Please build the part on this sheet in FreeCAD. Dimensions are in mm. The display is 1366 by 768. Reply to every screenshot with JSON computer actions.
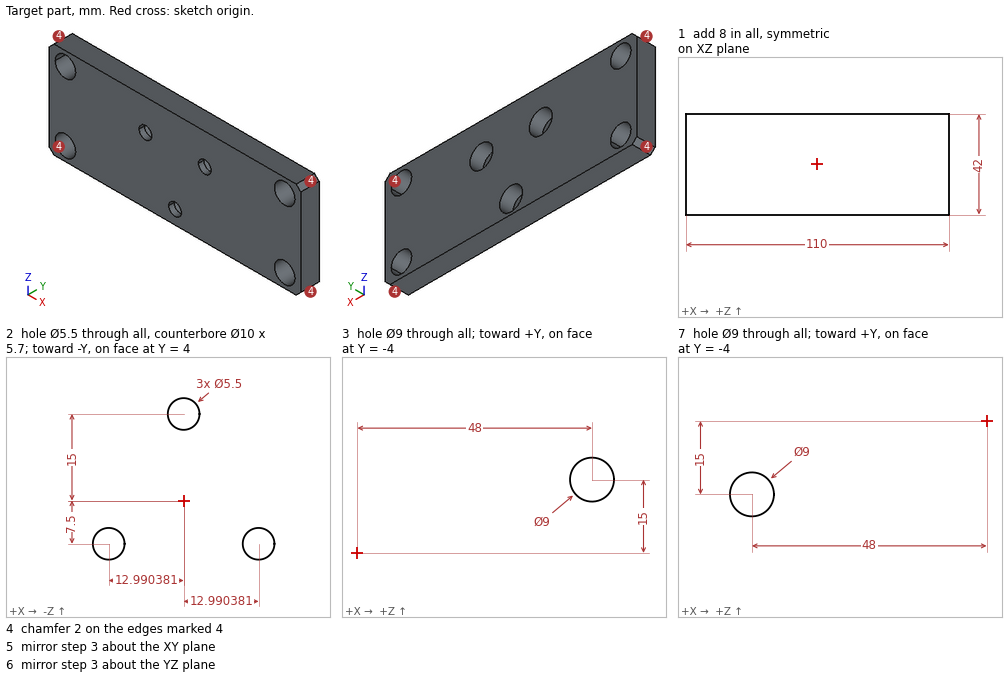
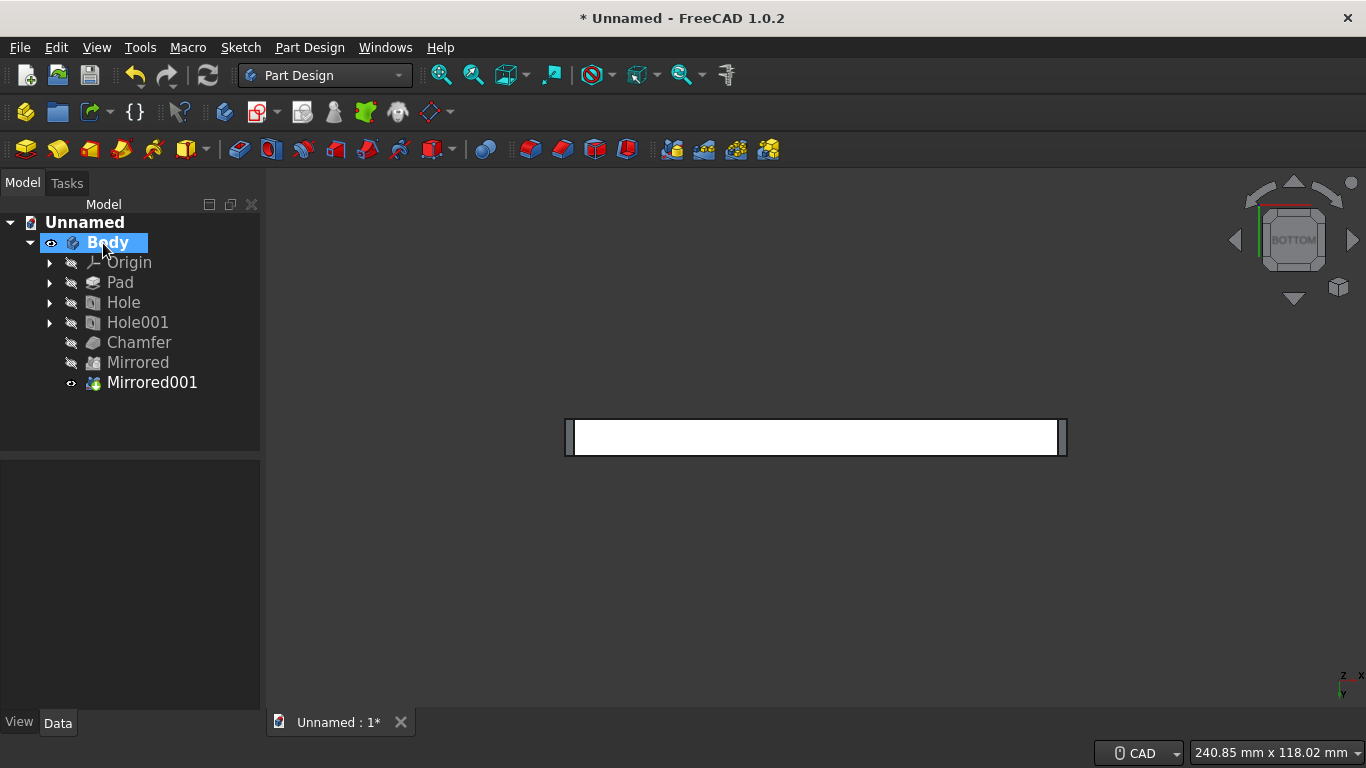
{"action": "key", "text": "0"}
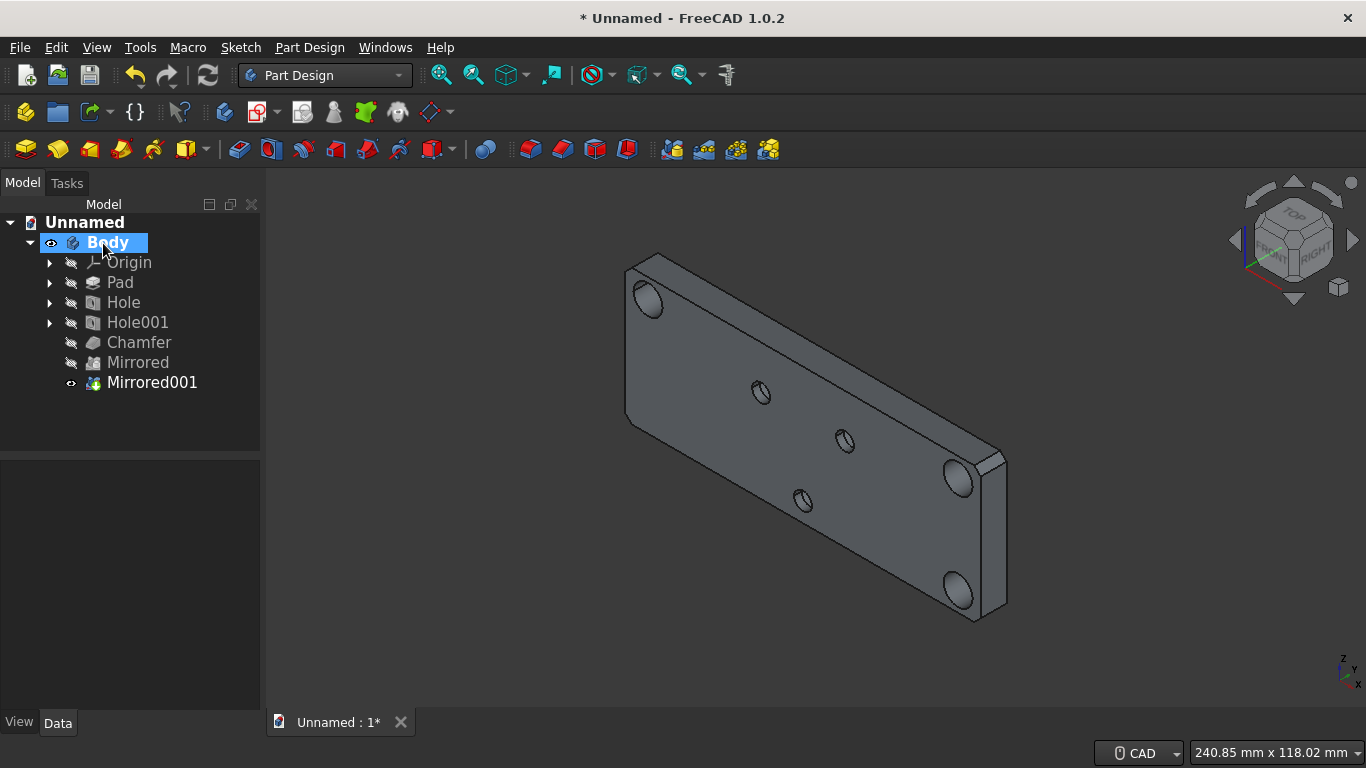
{"action": "left_click", "coordinate": [905, 503]}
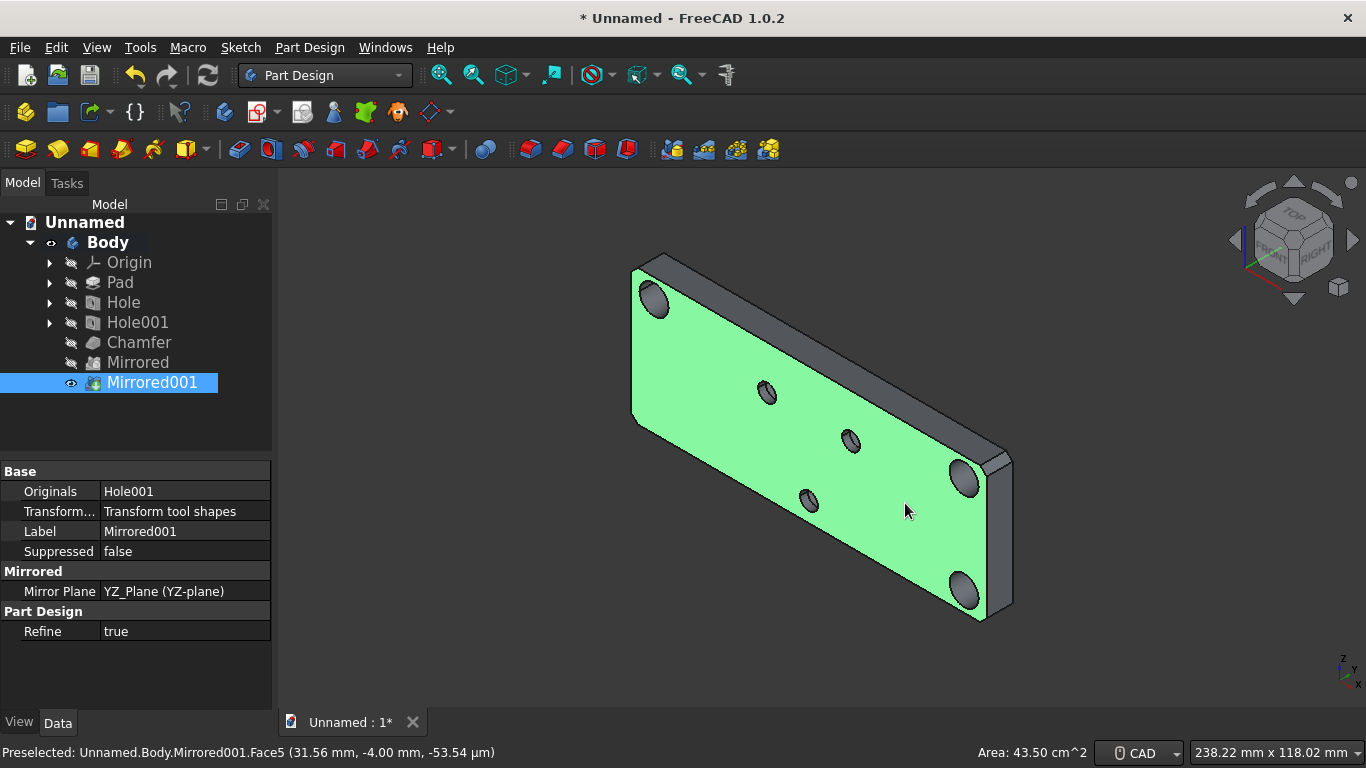
{"action": "left_click", "coordinate": [258, 112]}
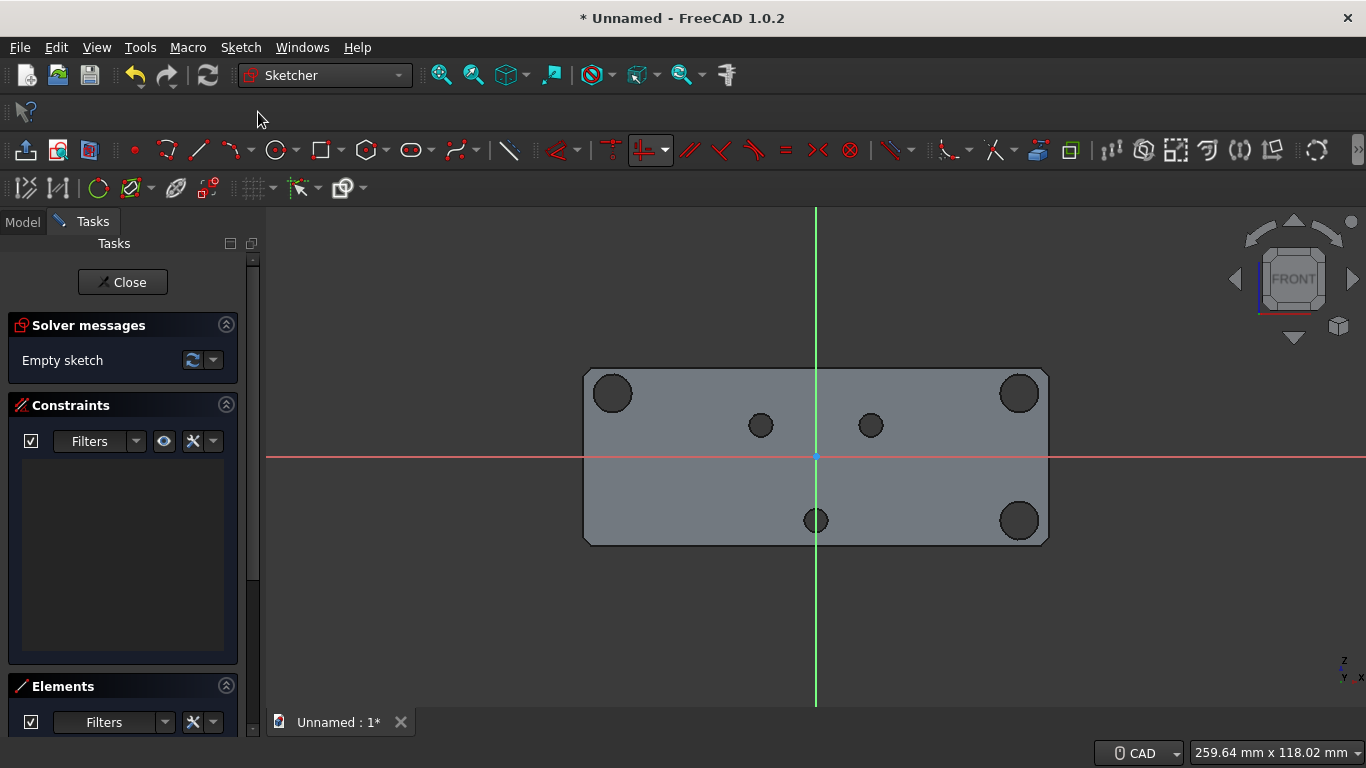
{"action": "scroll", "coordinate": [596, 528], "scroll_direction": "up", "scroll_amount": 11}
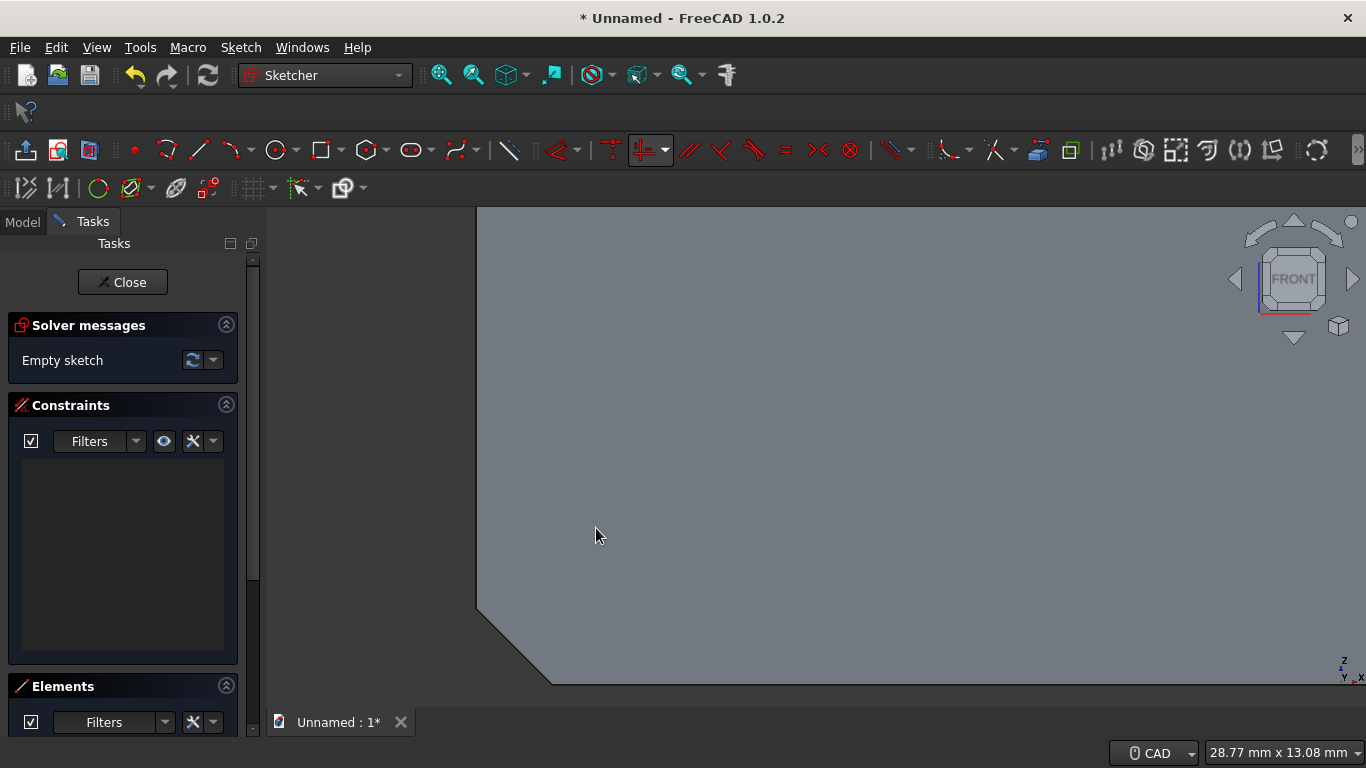
{"action": "left_click", "coordinate": [276, 150]}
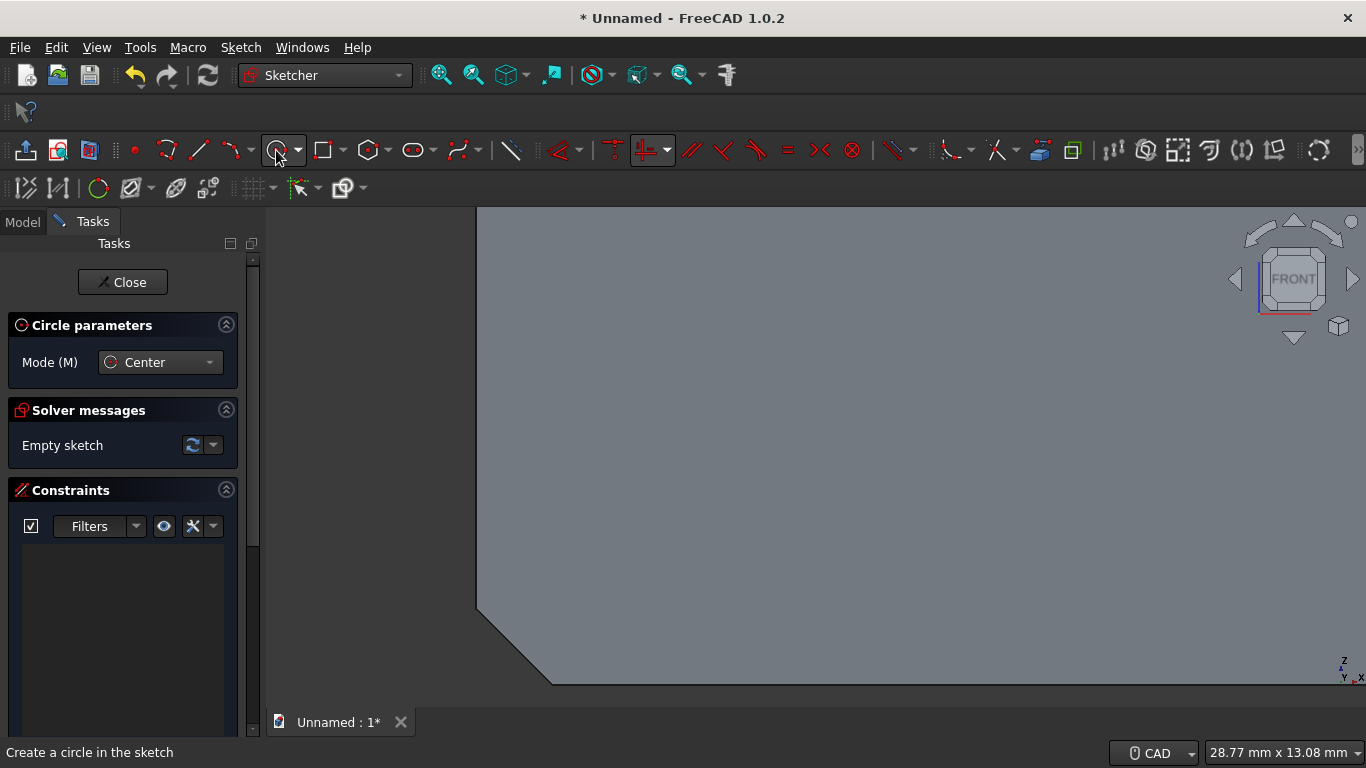
{"action": "left_click", "coordinate": [744, 456]}
{"action": "left_click", "coordinate": [865, 334]}
{"action": "key", "text": "Escape"}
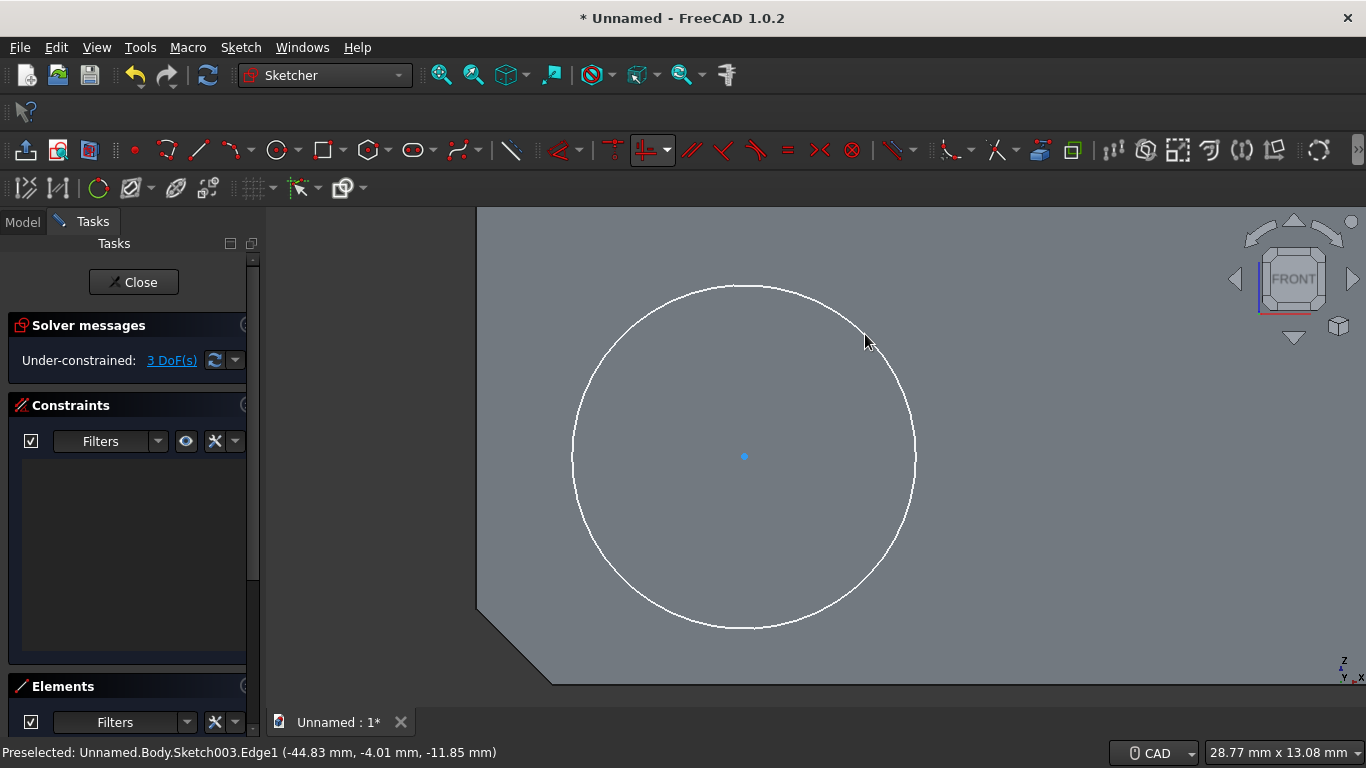
{"action": "left_click", "coordinate": [558, 150]}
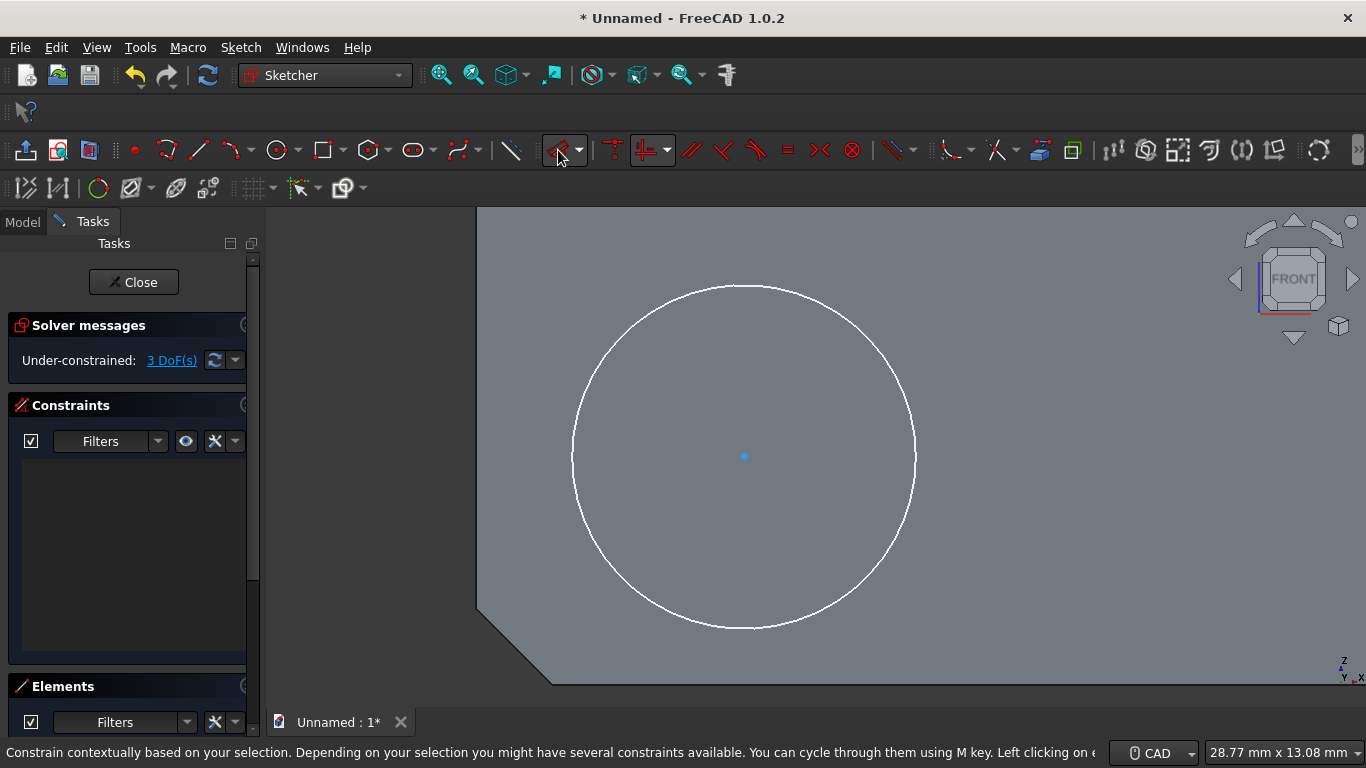
{"action": "left_click", "coordinate": [865, 335]}
{"action": "left_click", "coordinate": [888, 312]}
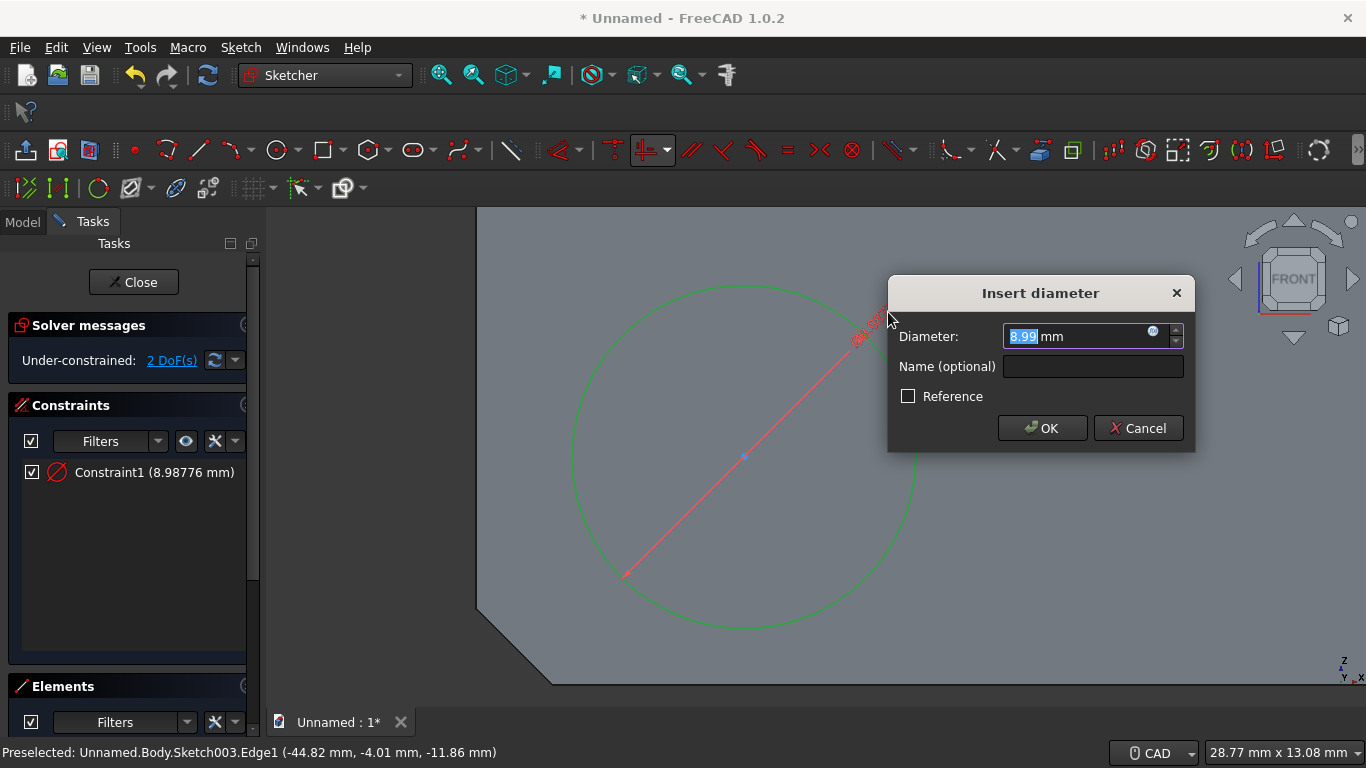
{"action": "type", "text": "9"}
{"action": "key", "text": "Return"}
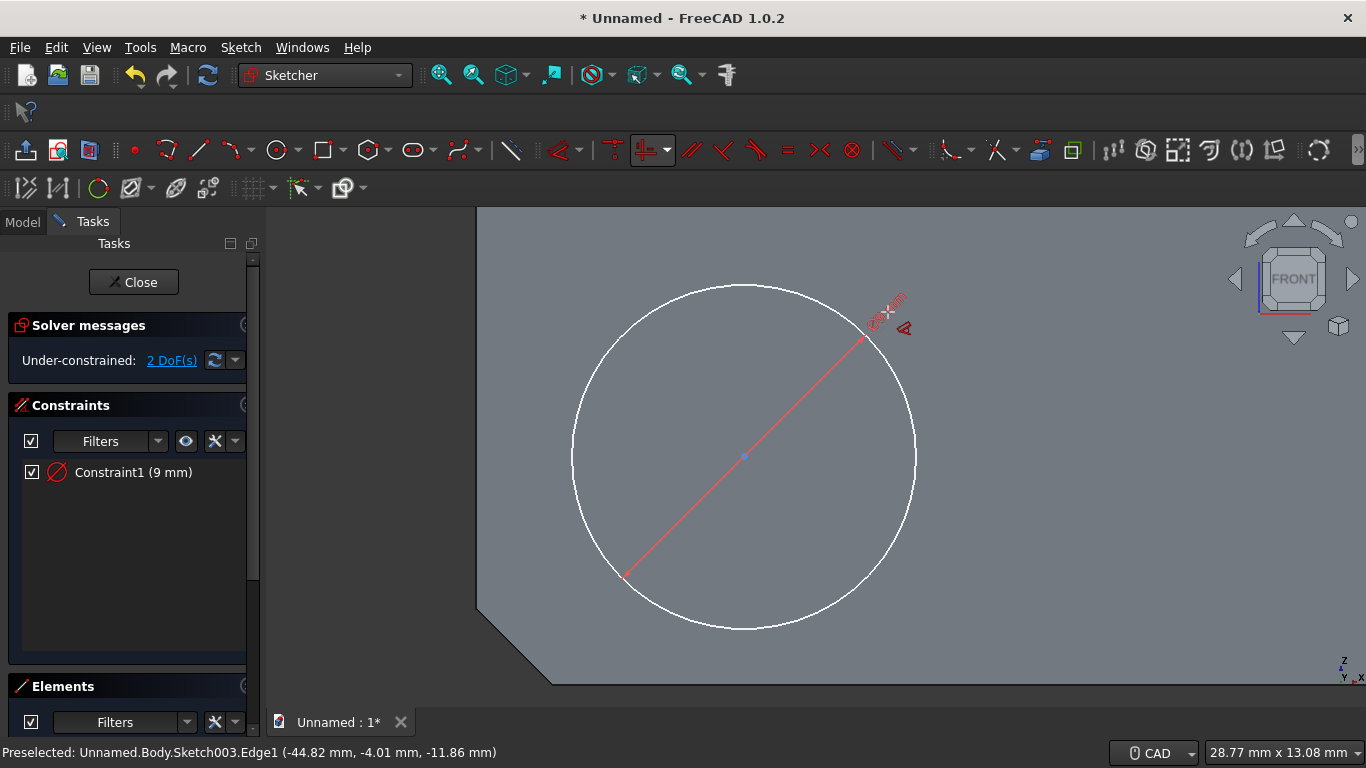
{"action": "left_click", "coordinate": [744, 457]}
{"action": "left_click", "coordinate": [973, 491]}